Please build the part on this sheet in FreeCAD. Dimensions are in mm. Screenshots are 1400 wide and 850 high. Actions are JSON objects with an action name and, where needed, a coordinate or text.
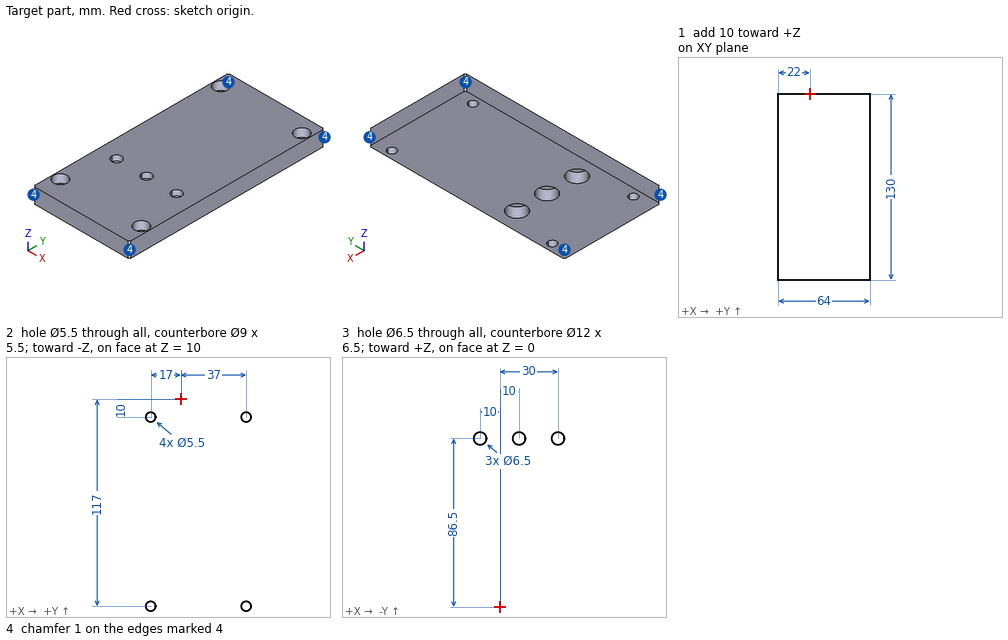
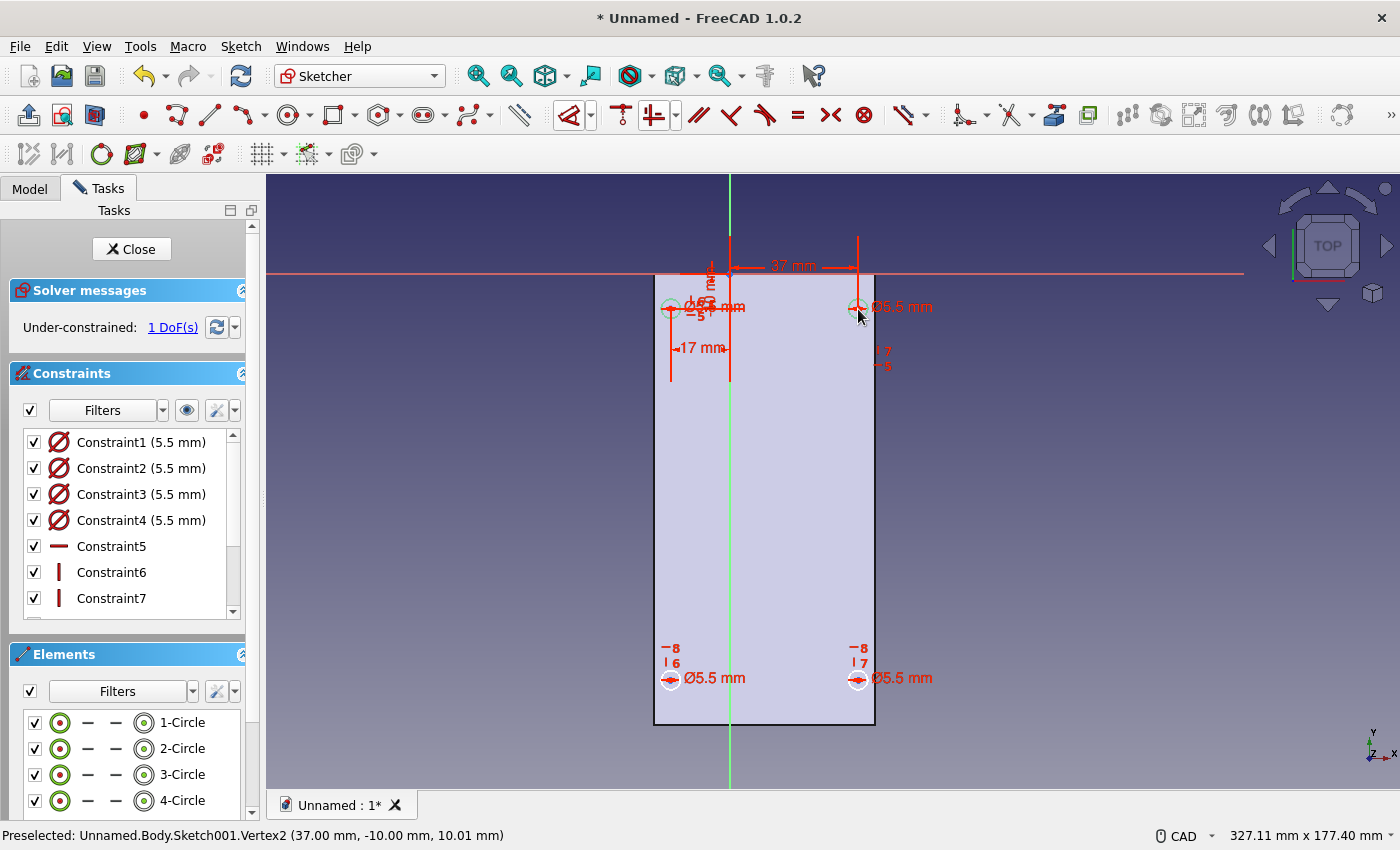
{"action": "left_click", "coordinate": [671, 680]}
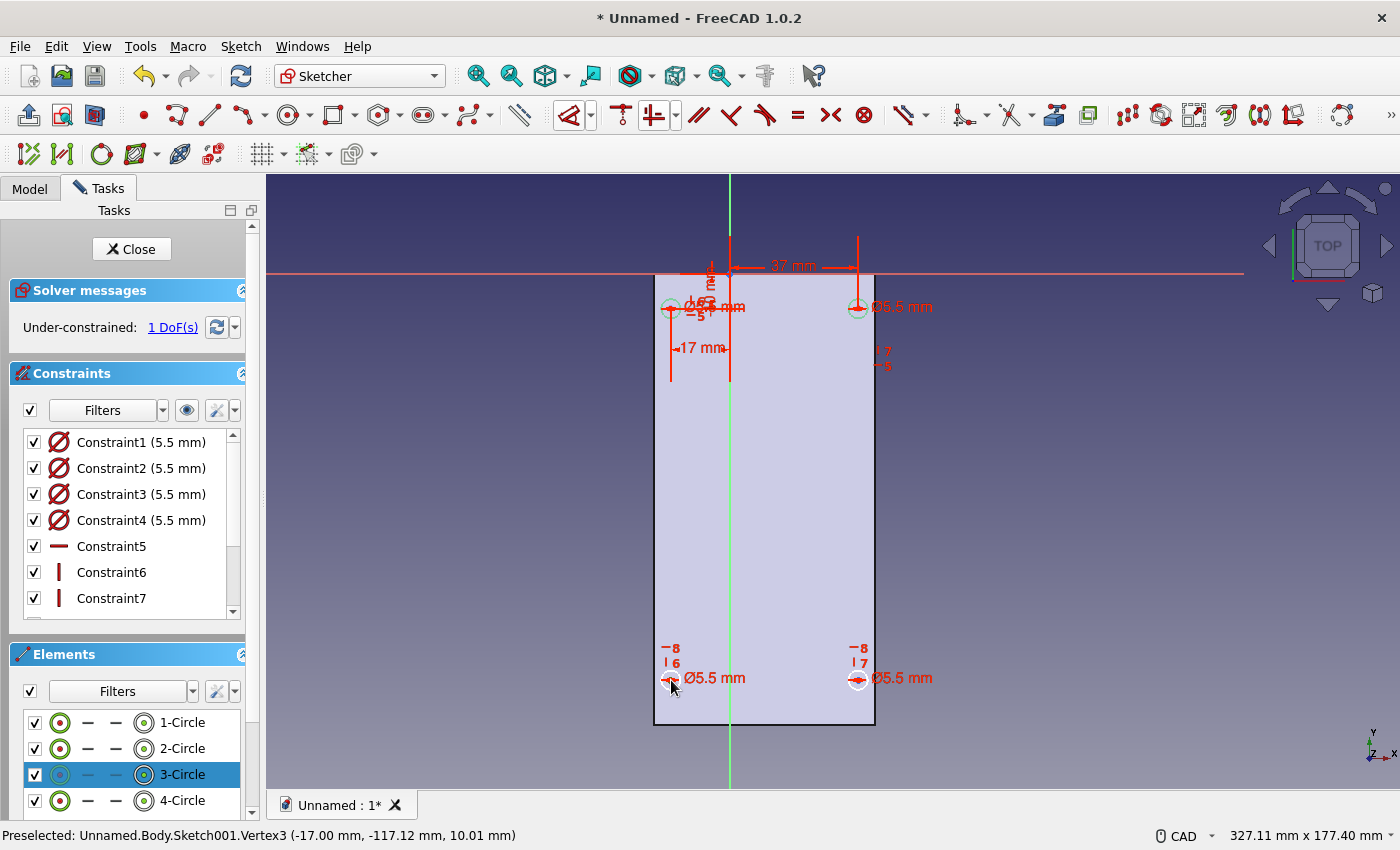
{"action": "key", "text": "i"}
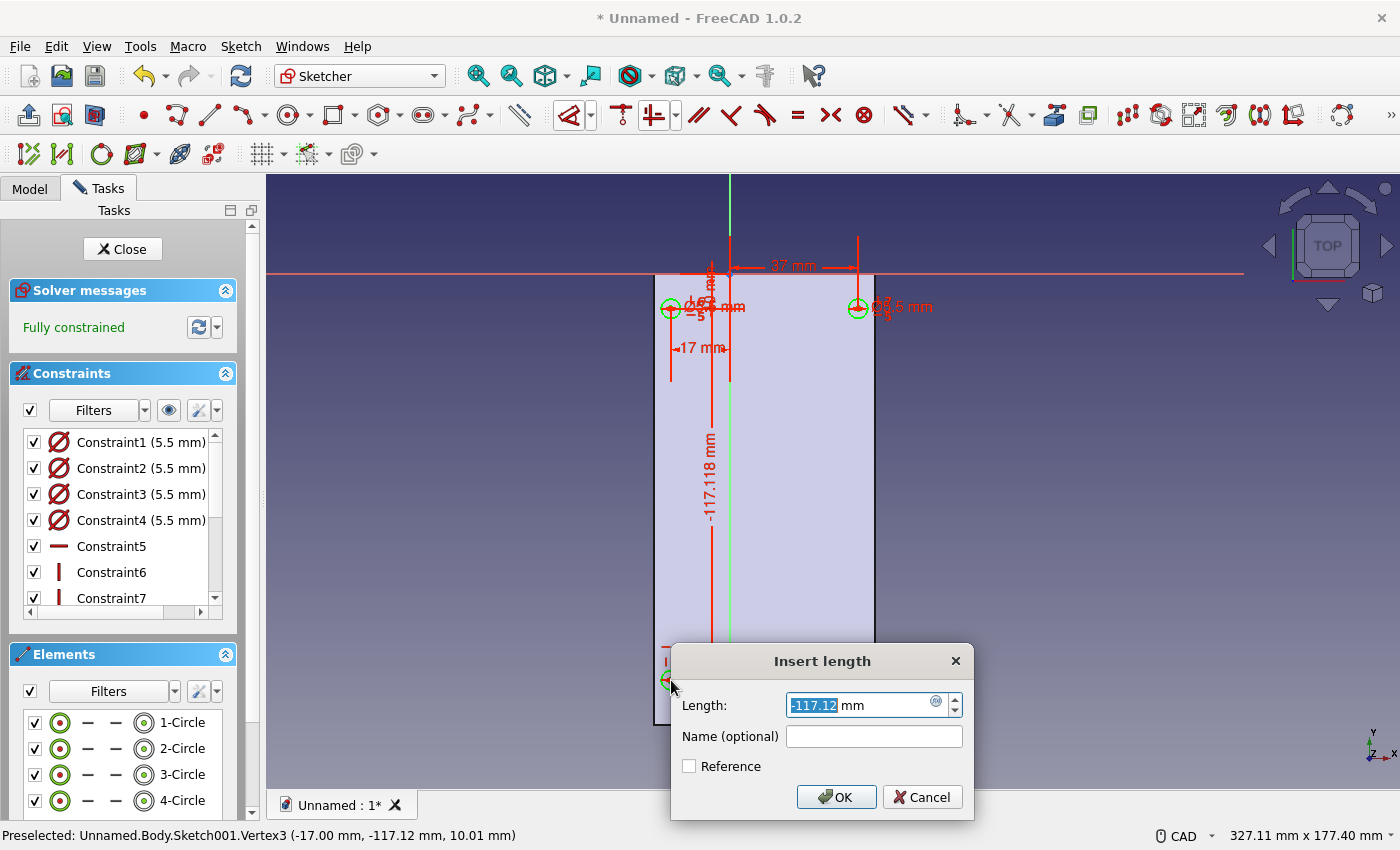
{"action": "type", "text": "-117"}
{"action": "key", "text": "Return"}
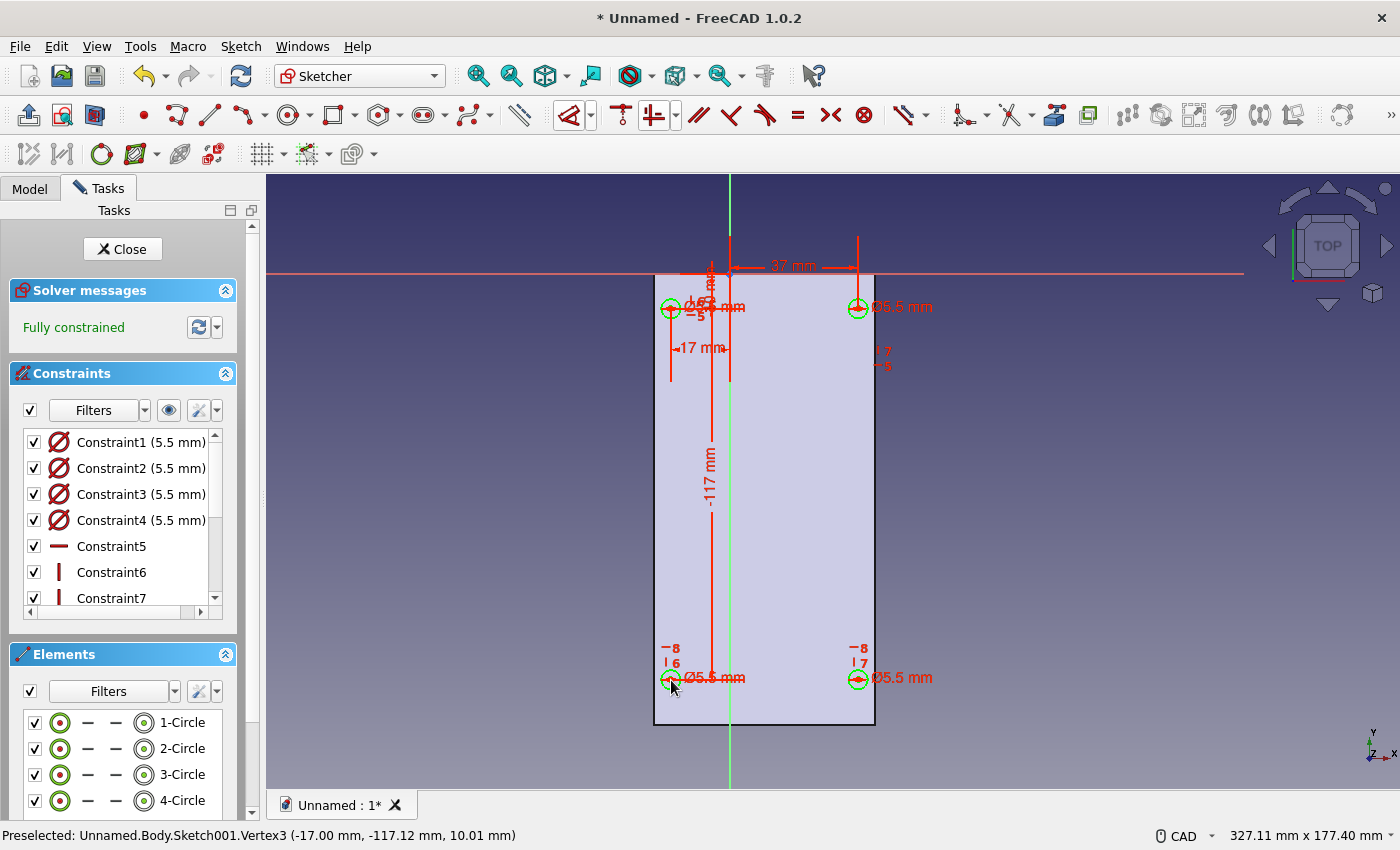
{"action": "left_click", "coordinate": [123, 249]}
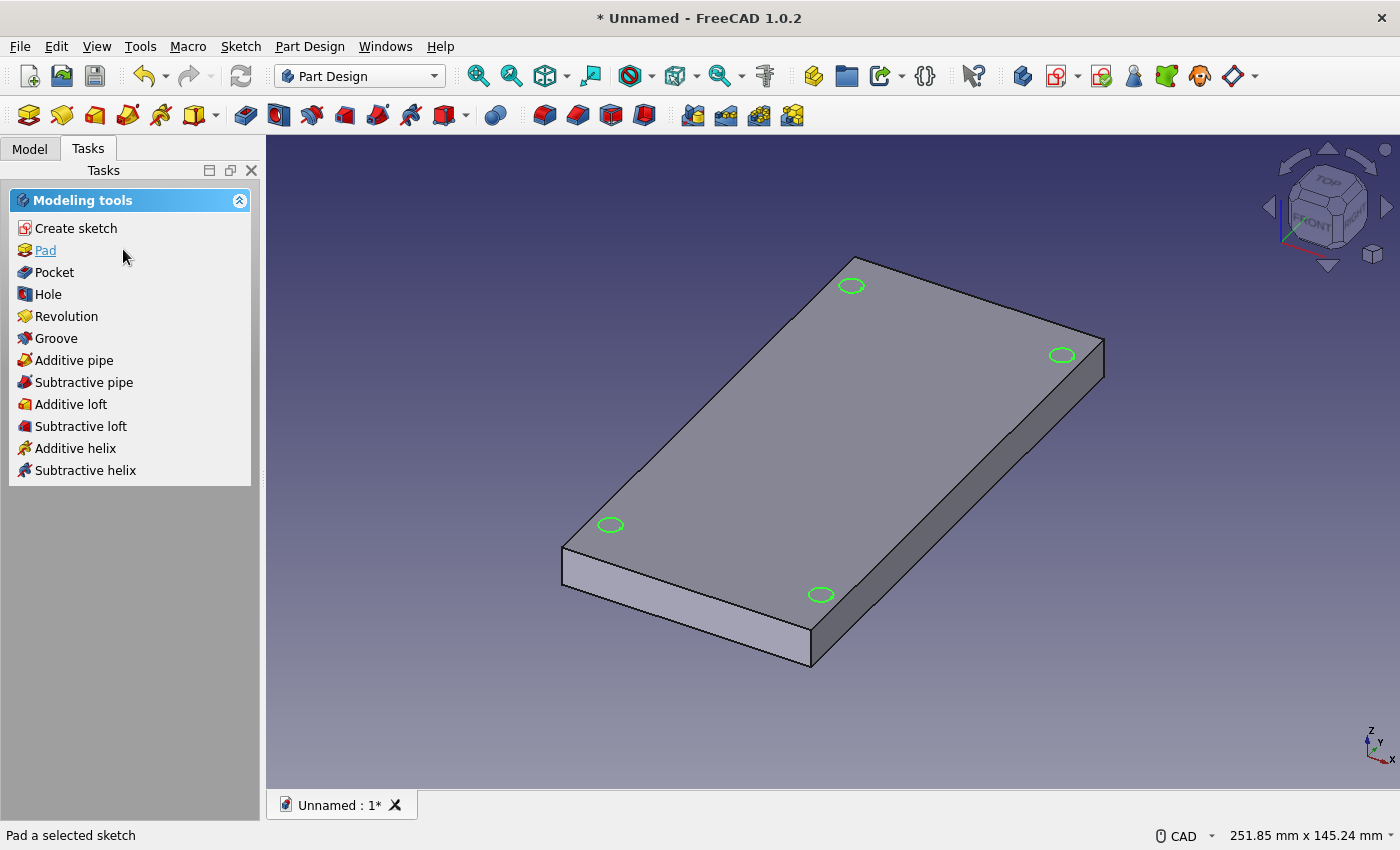
{"action": "left_click", "coordinate": [279, 116]}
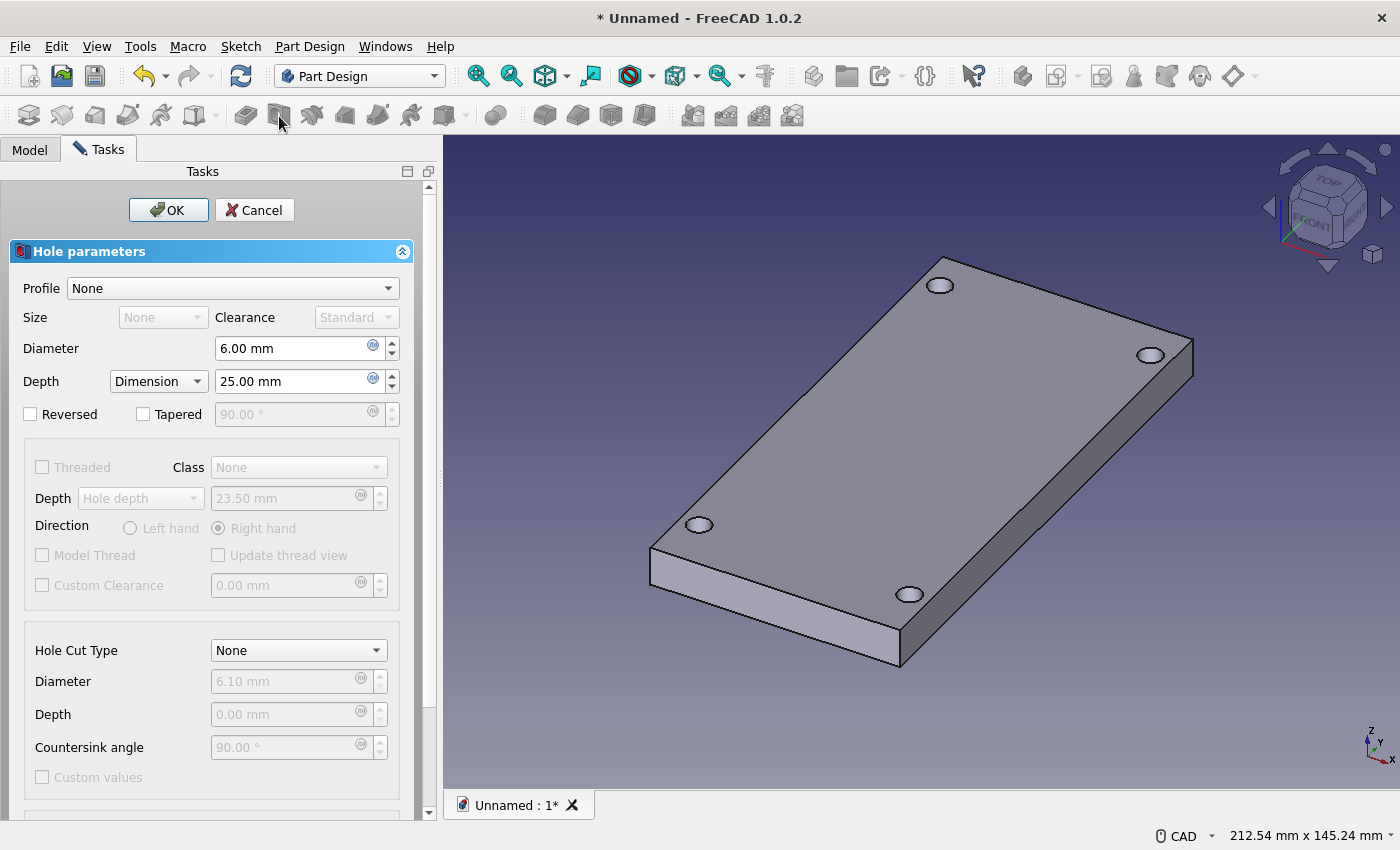
{"action": "triple_click", "coordinate": [300, 348]}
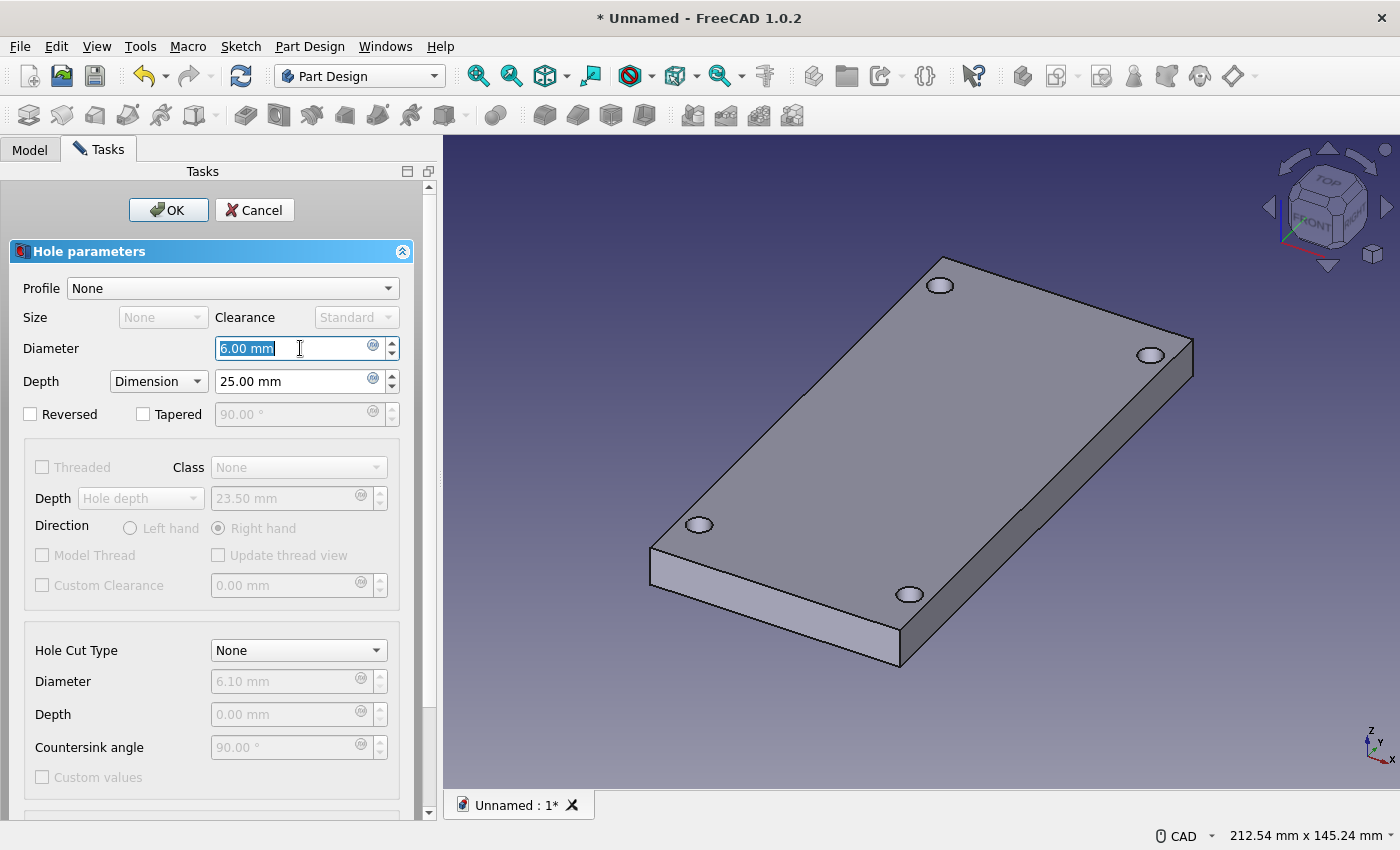
{"action": "type", "text": "5.5"}
{"action": "key", "text": "Tab"}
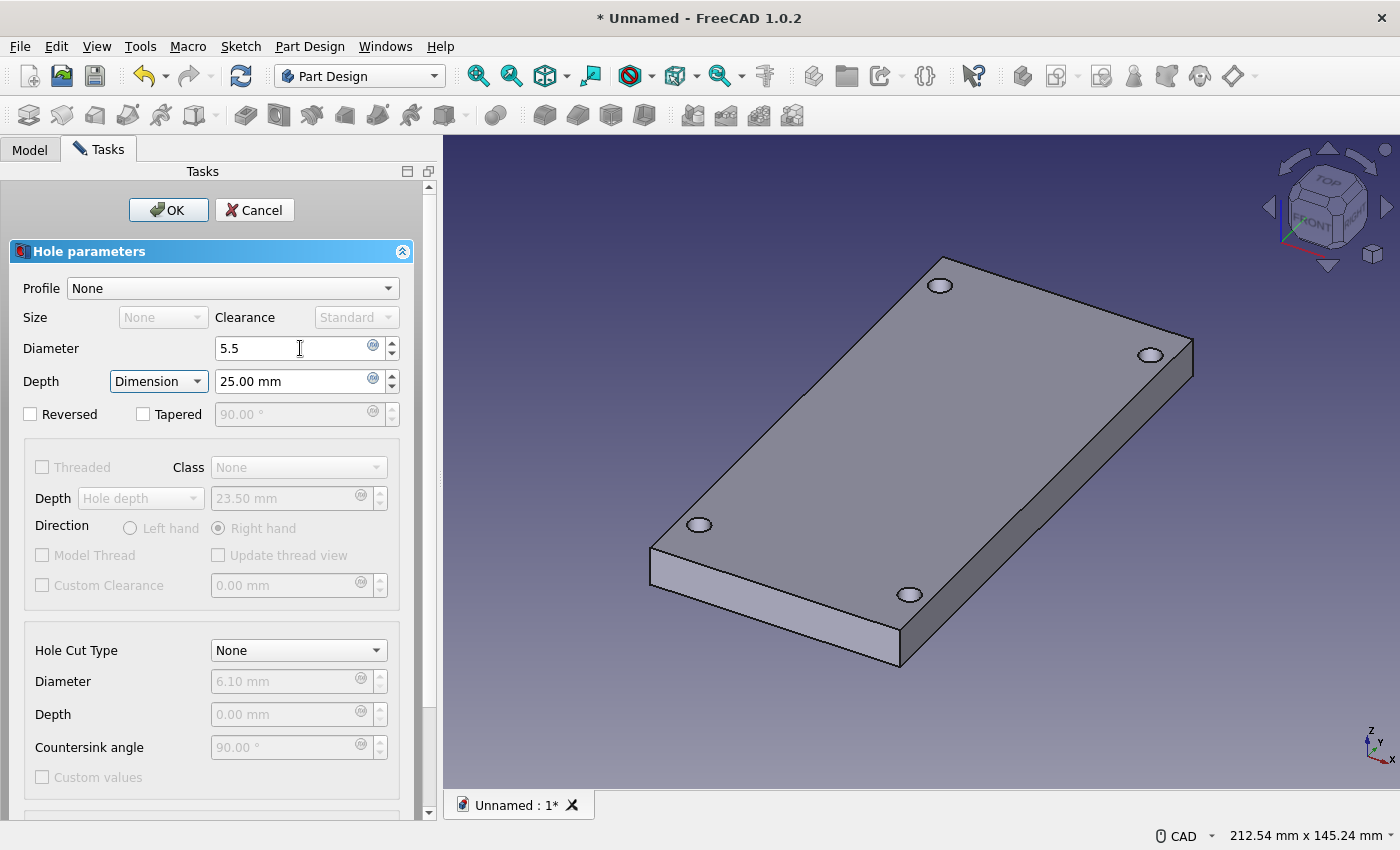
{"action": "left_click", "coordinate": [160, 382]}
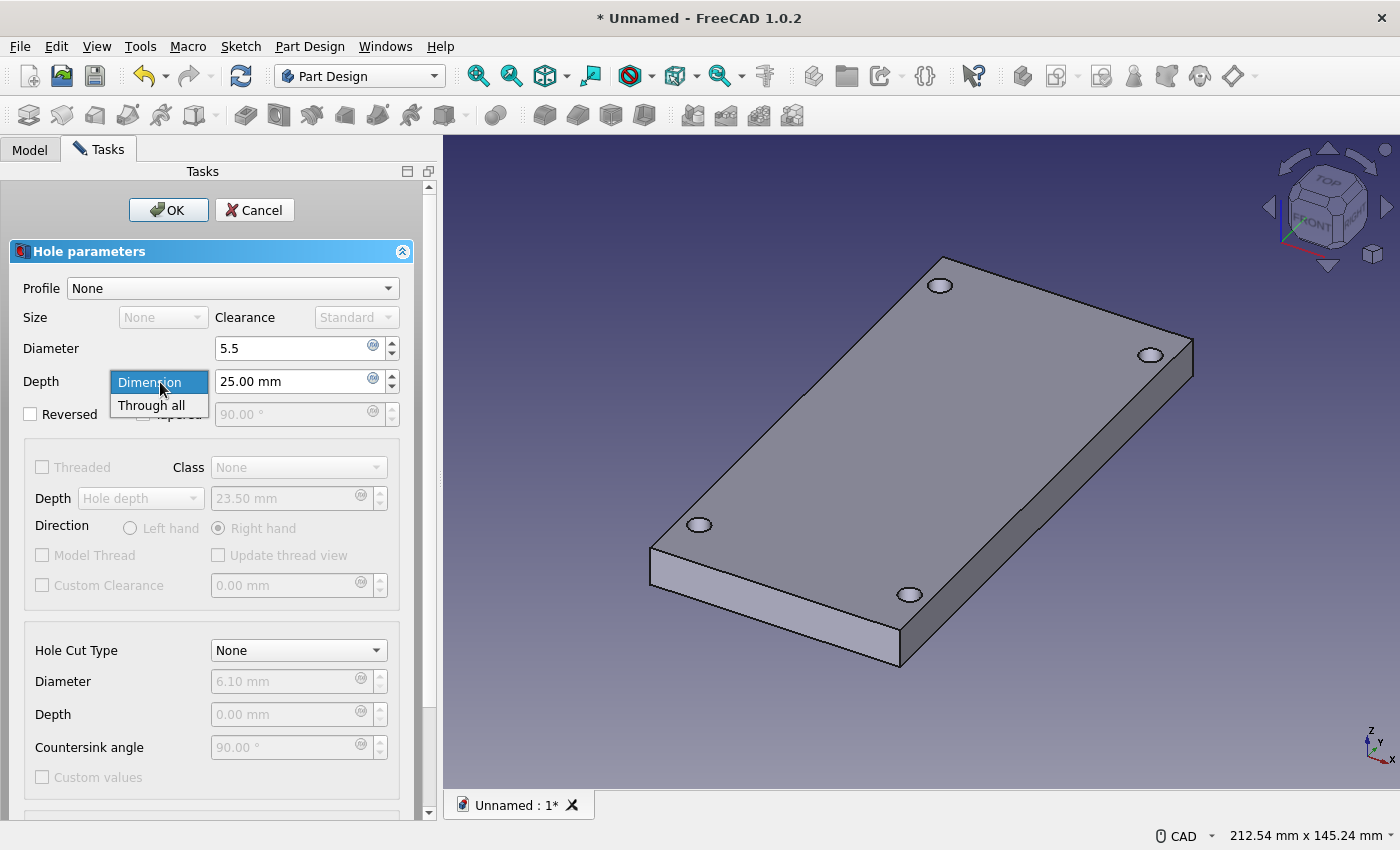
{"action": "left_click", "coordinate": [158, 406]}